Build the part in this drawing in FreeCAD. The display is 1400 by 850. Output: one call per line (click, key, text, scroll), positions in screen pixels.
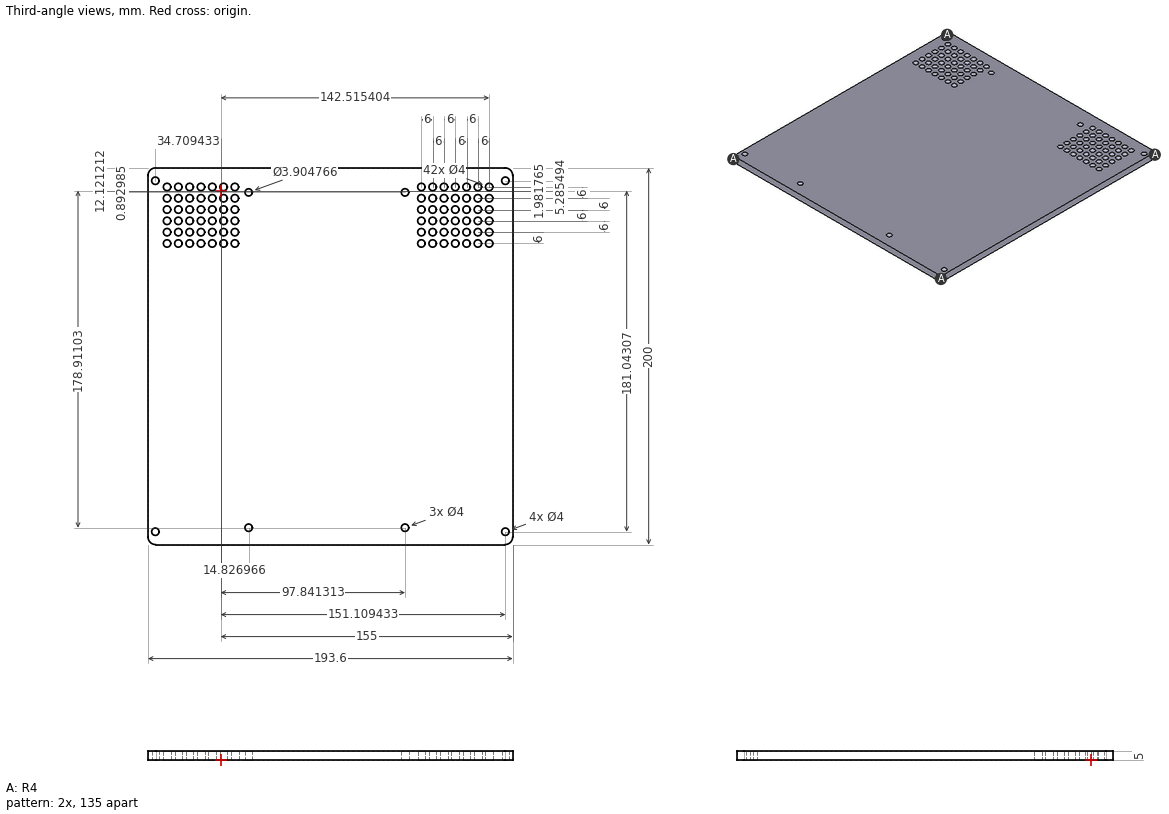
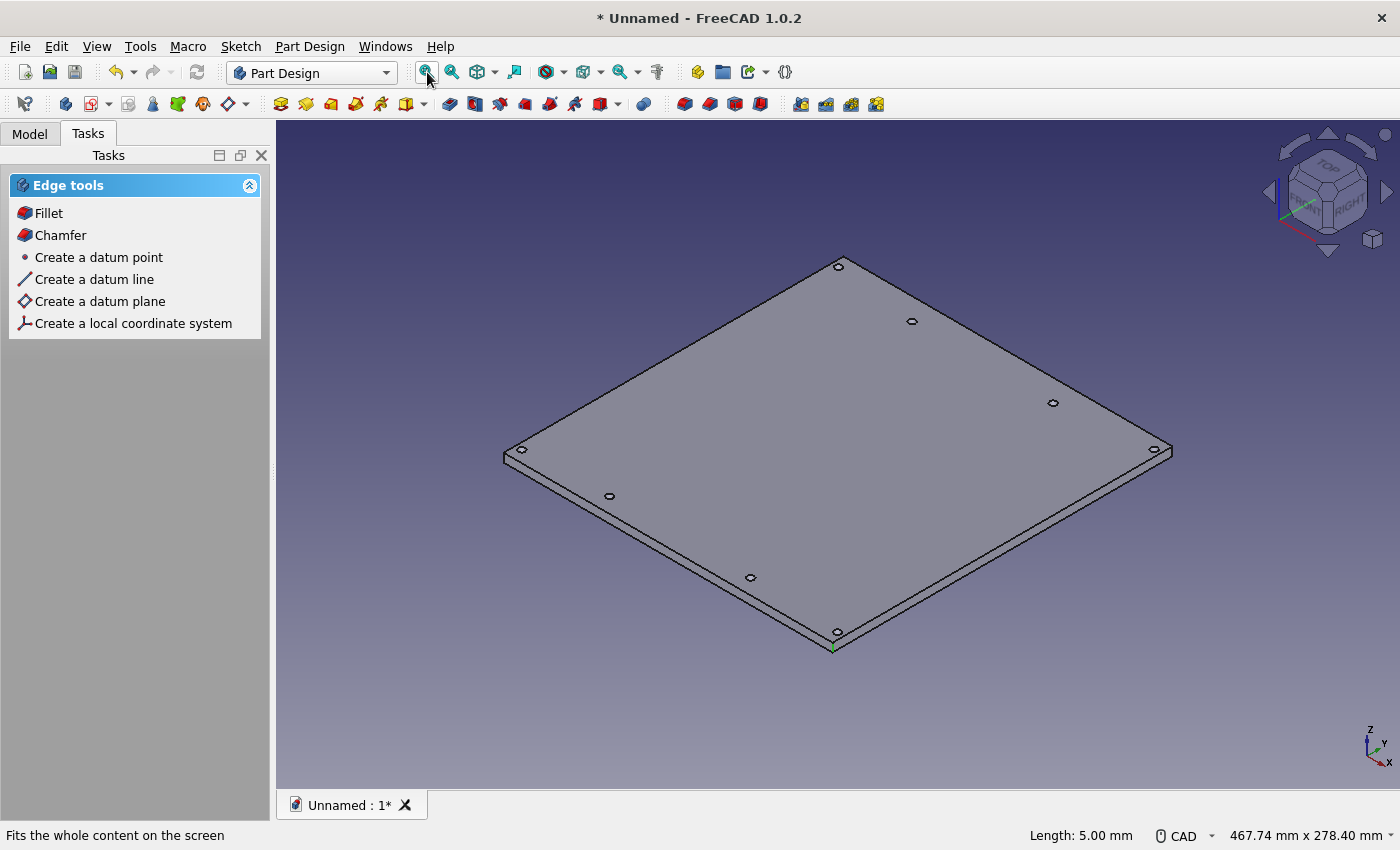
key(2)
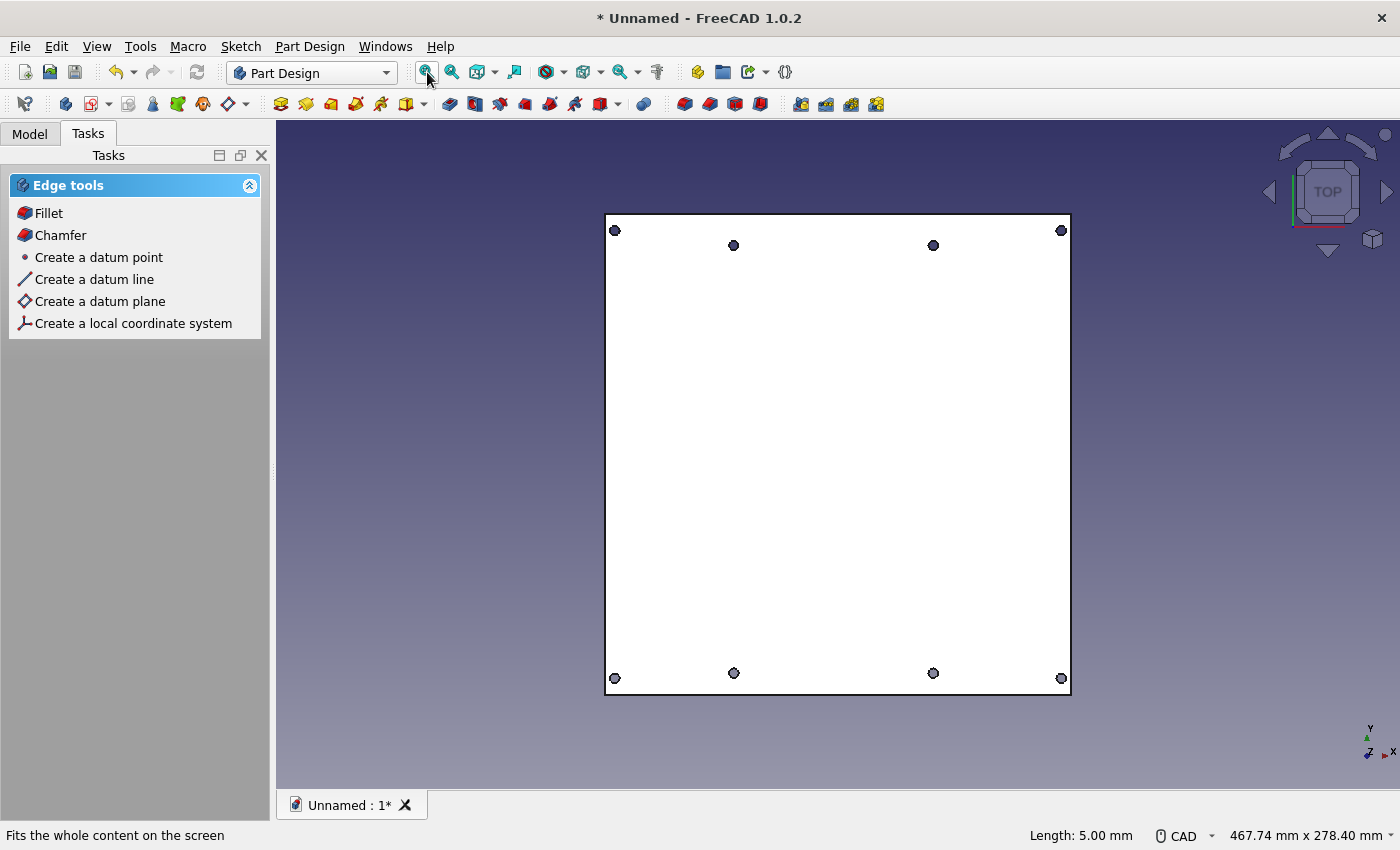
scroll(605, 213, up, 7)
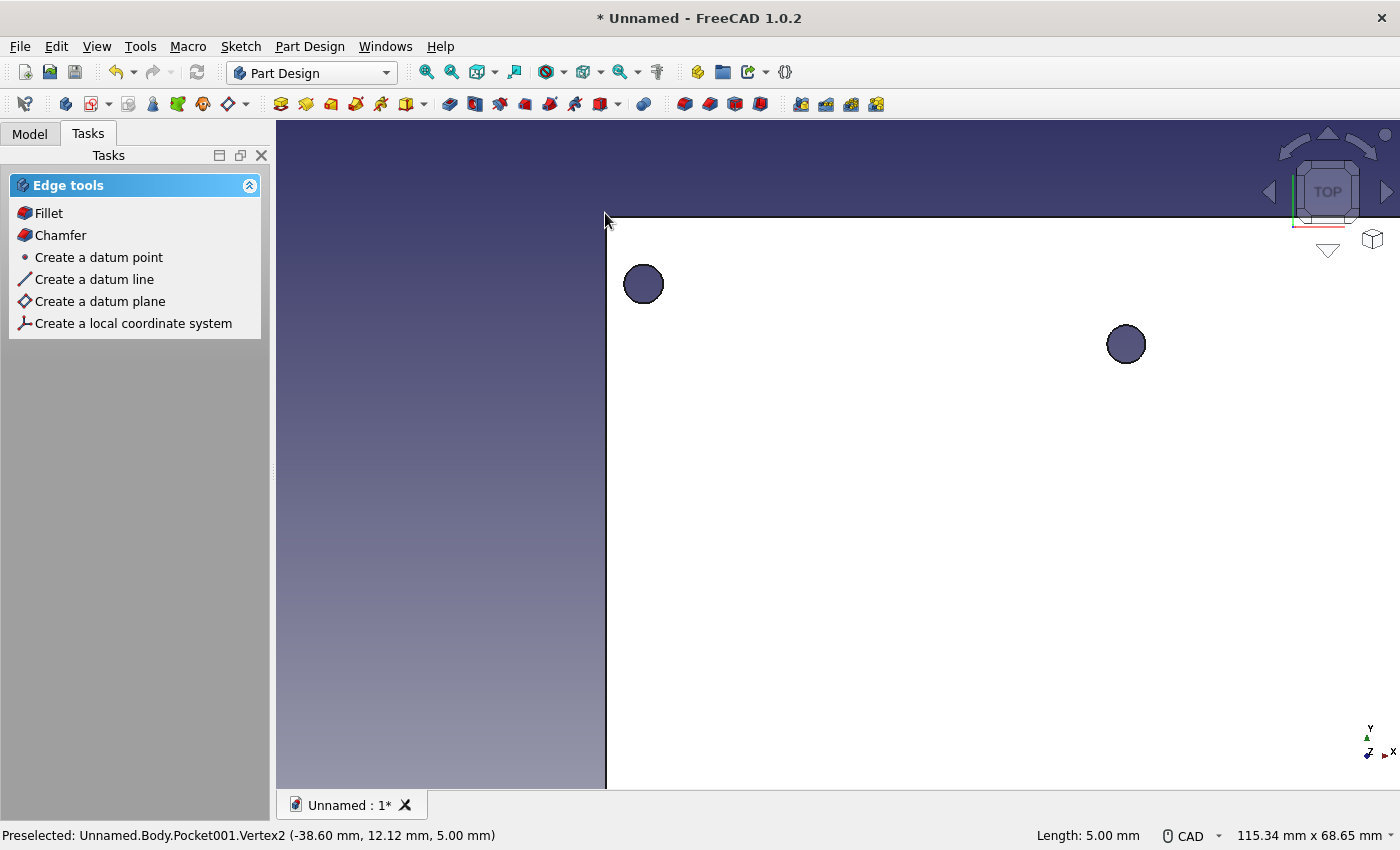
click(427, 72)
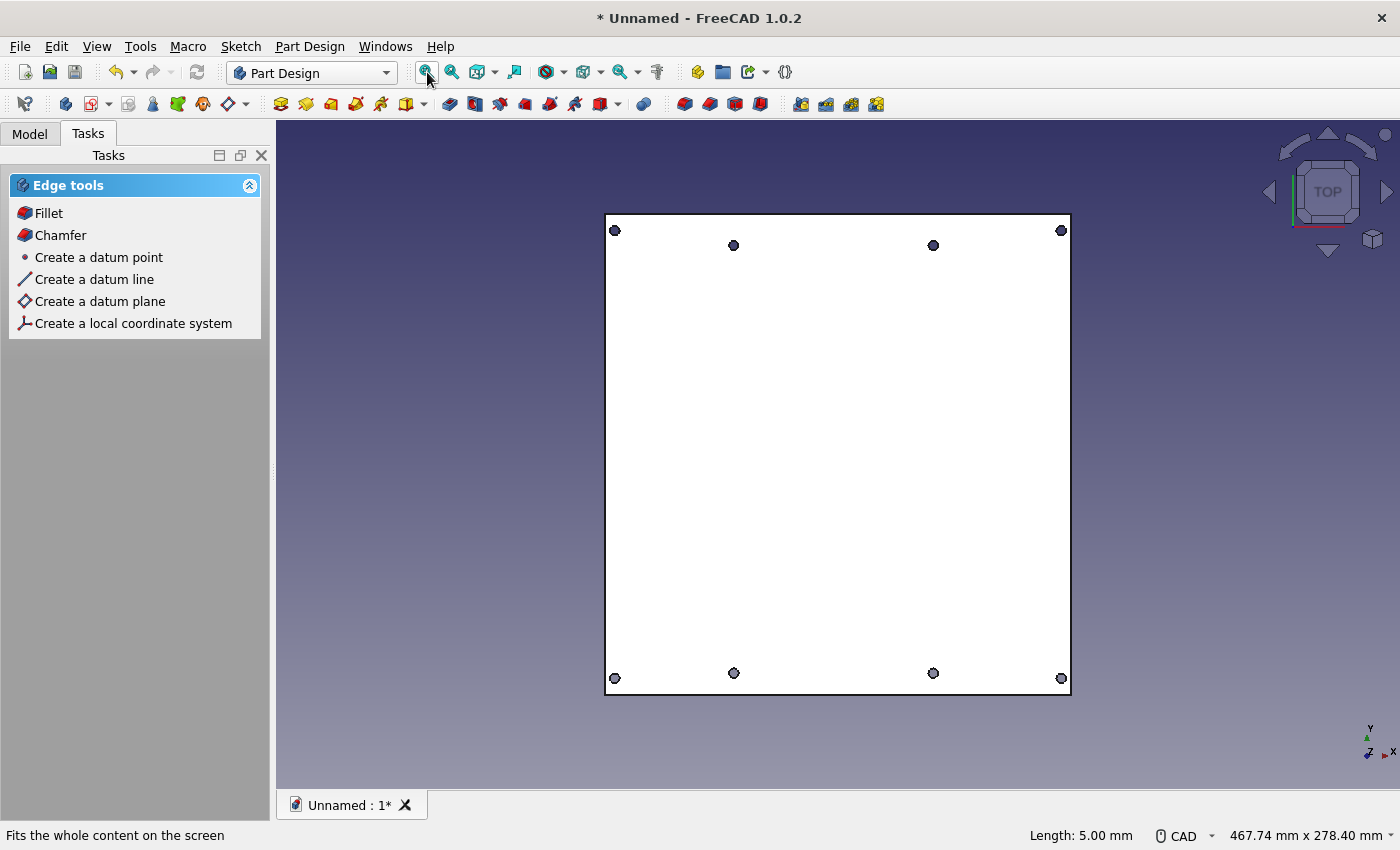
key(1)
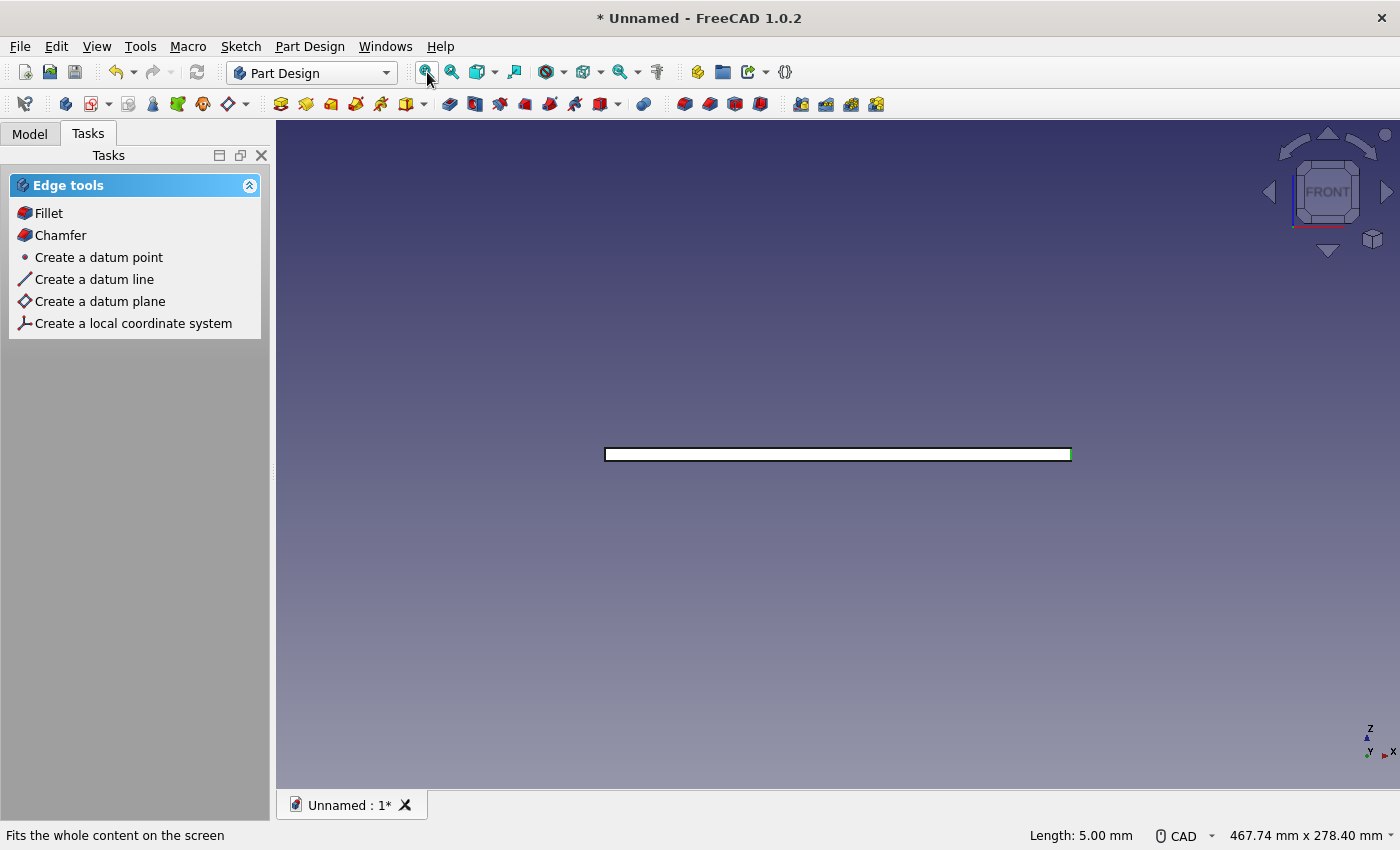
click(427, 72)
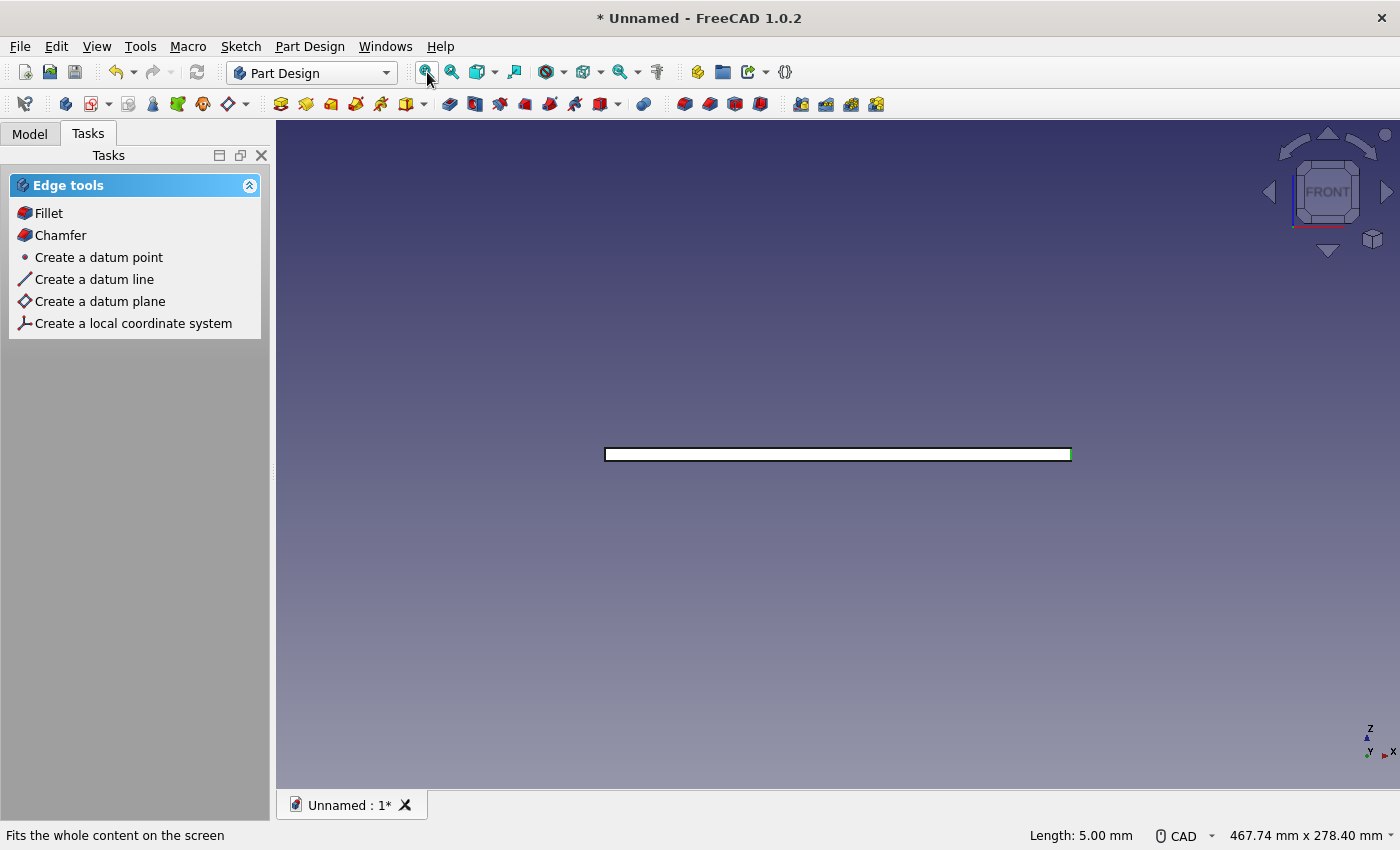
scroll(605, 454, up, 7)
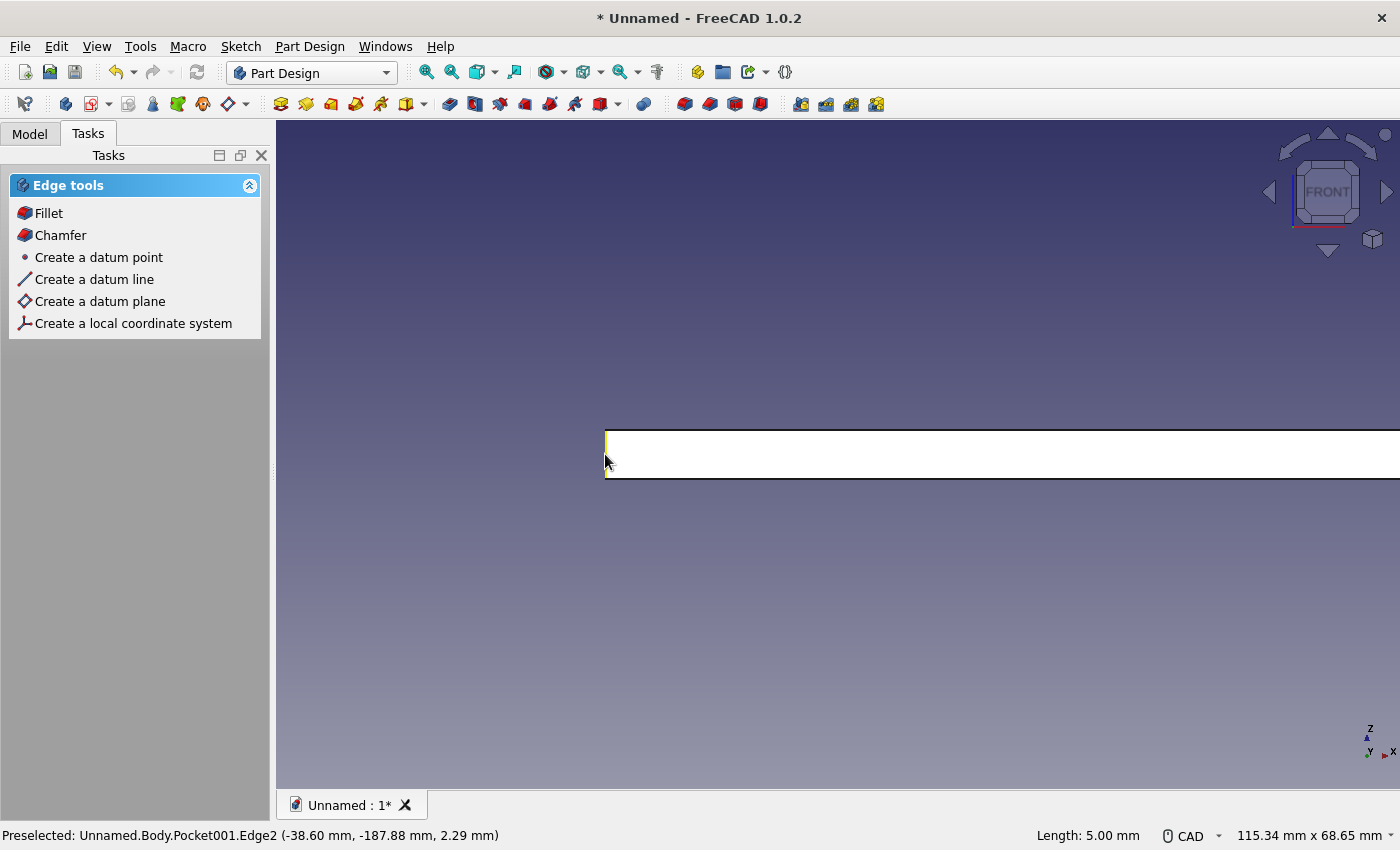
click(606, 454, ctrl)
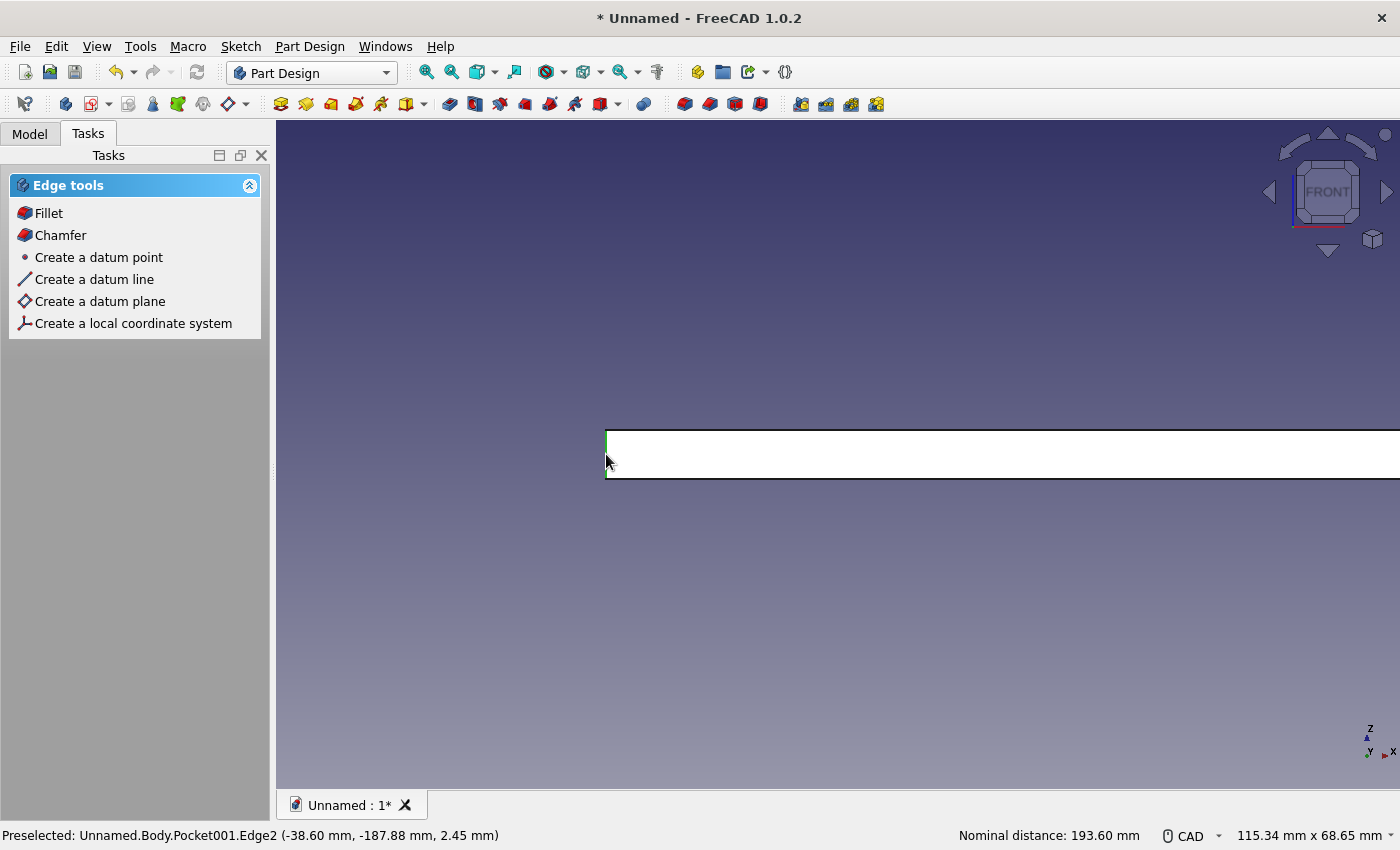
click(427, 72)